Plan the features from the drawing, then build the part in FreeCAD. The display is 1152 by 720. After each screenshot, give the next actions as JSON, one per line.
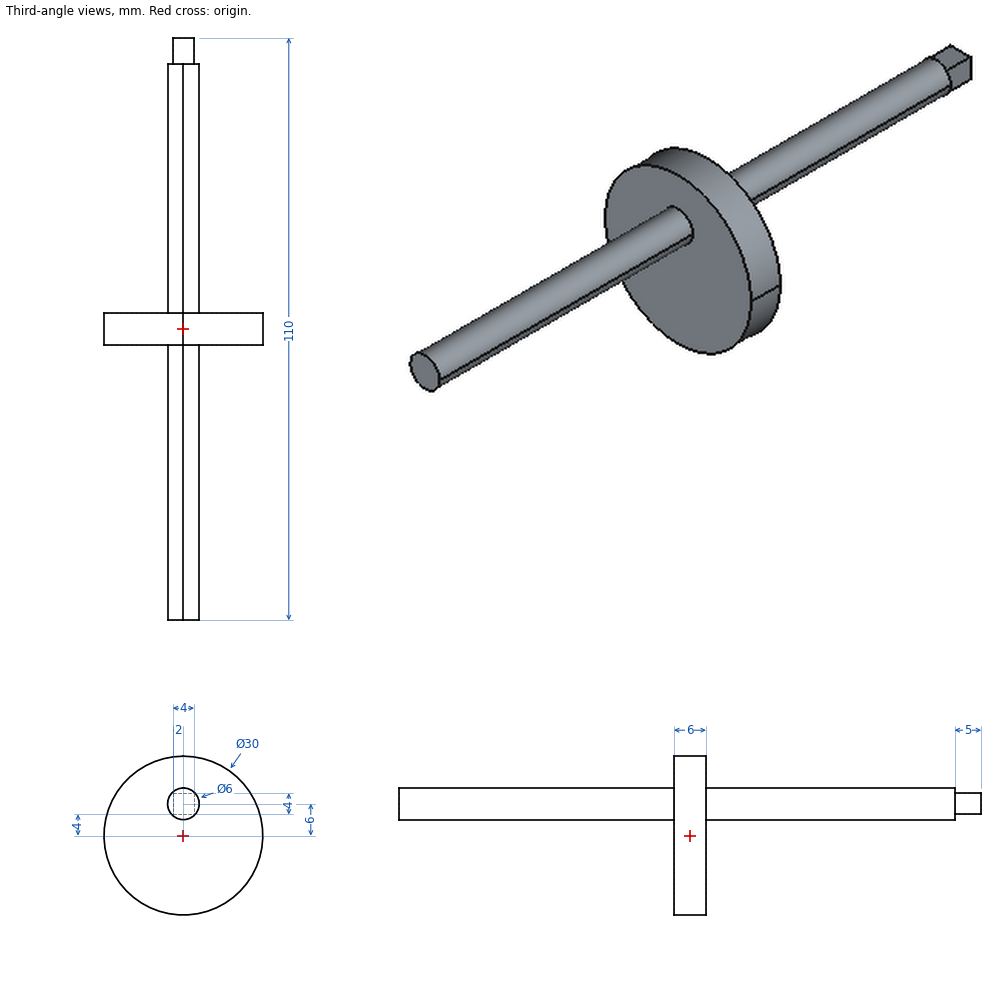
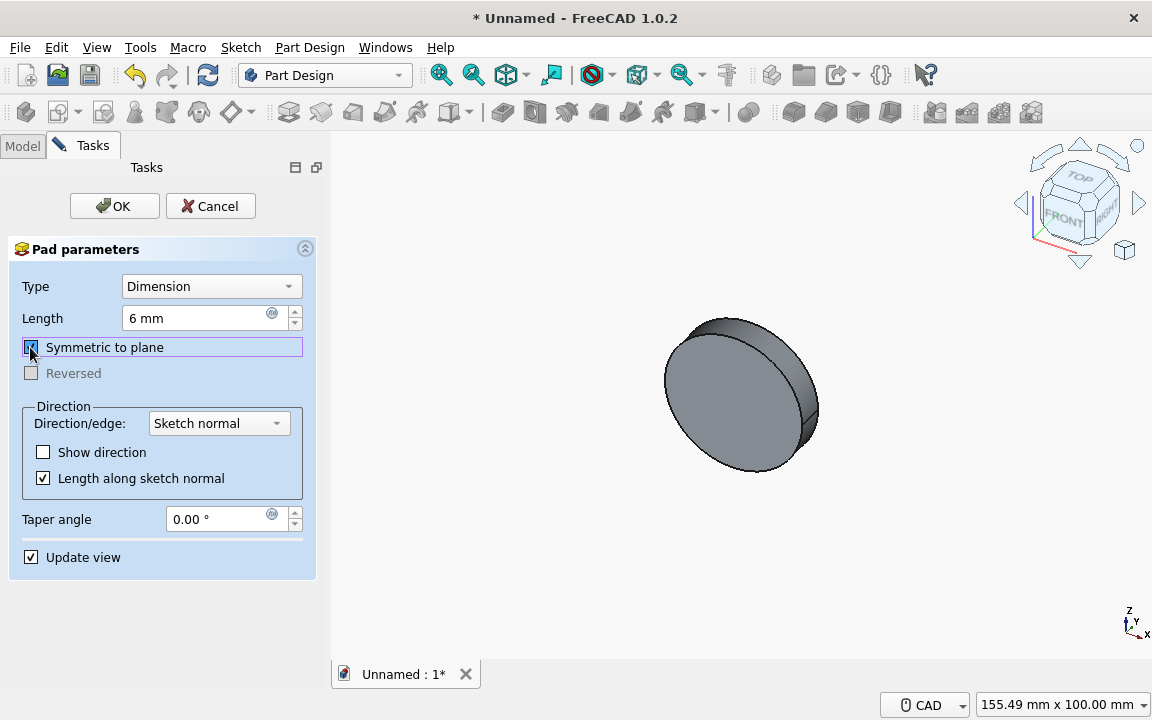
{"action": "left_click", "coordinate": [115, 206]}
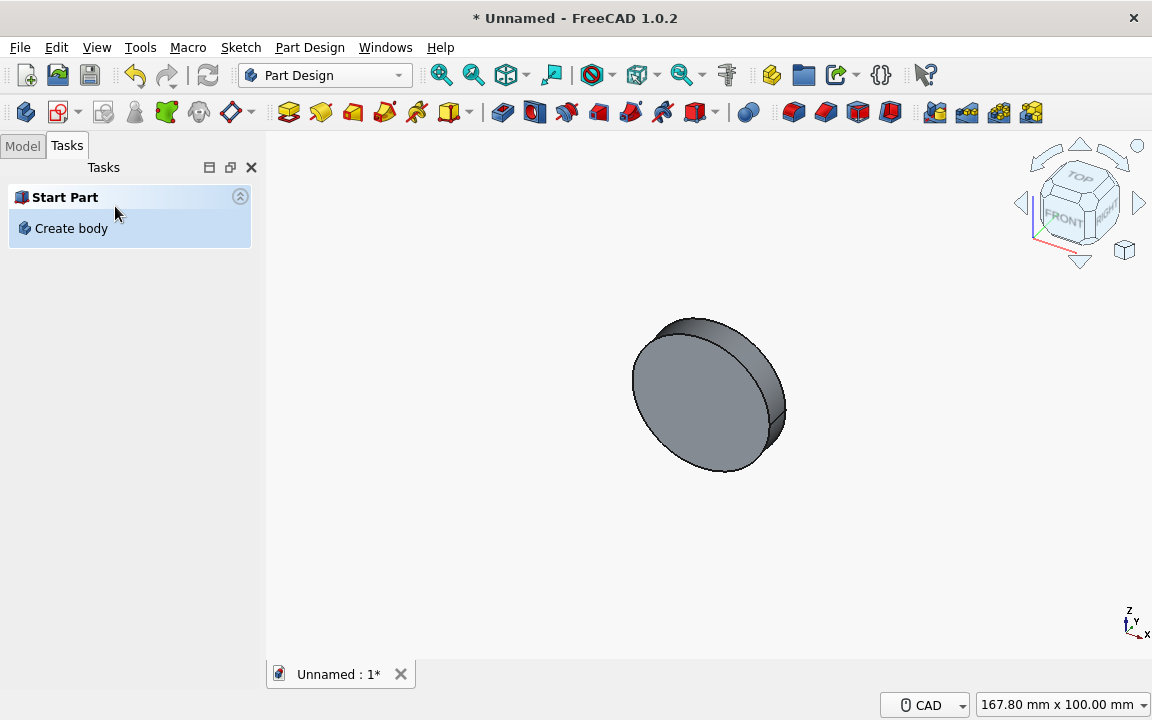
{"action": "key", "text": "v f"}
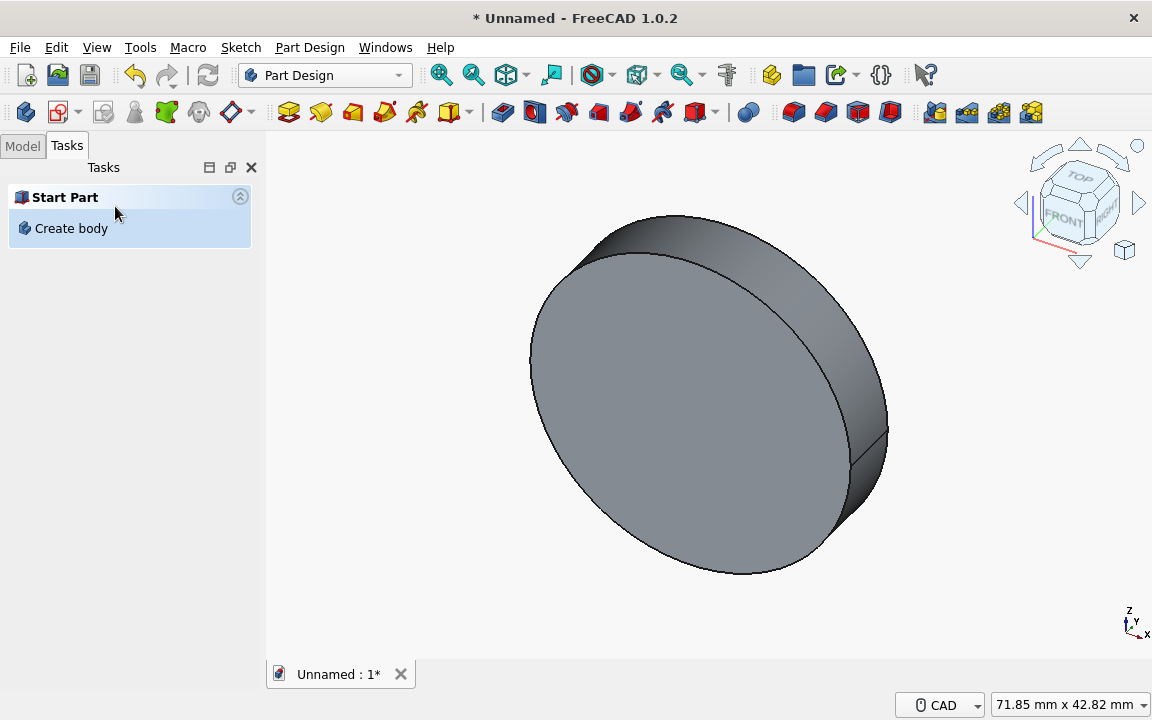
{"action": "left_click", "coordinate": [58, 112]}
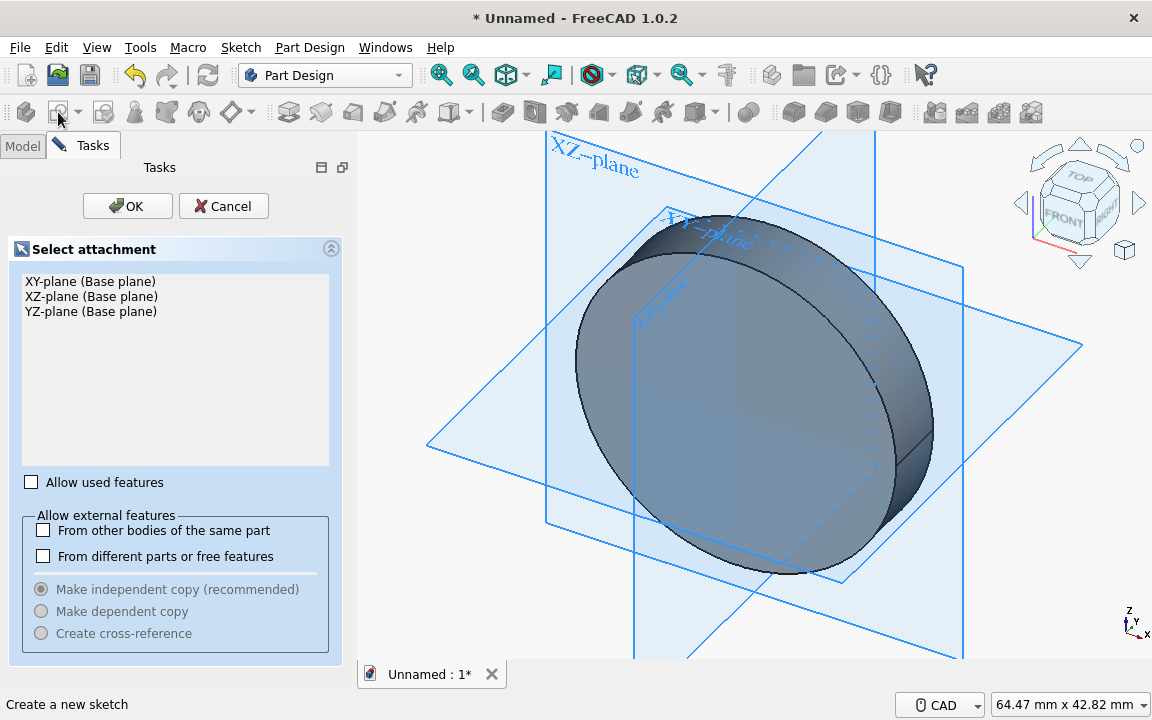
{"action": "left_click", "coordinate": [82, 296]}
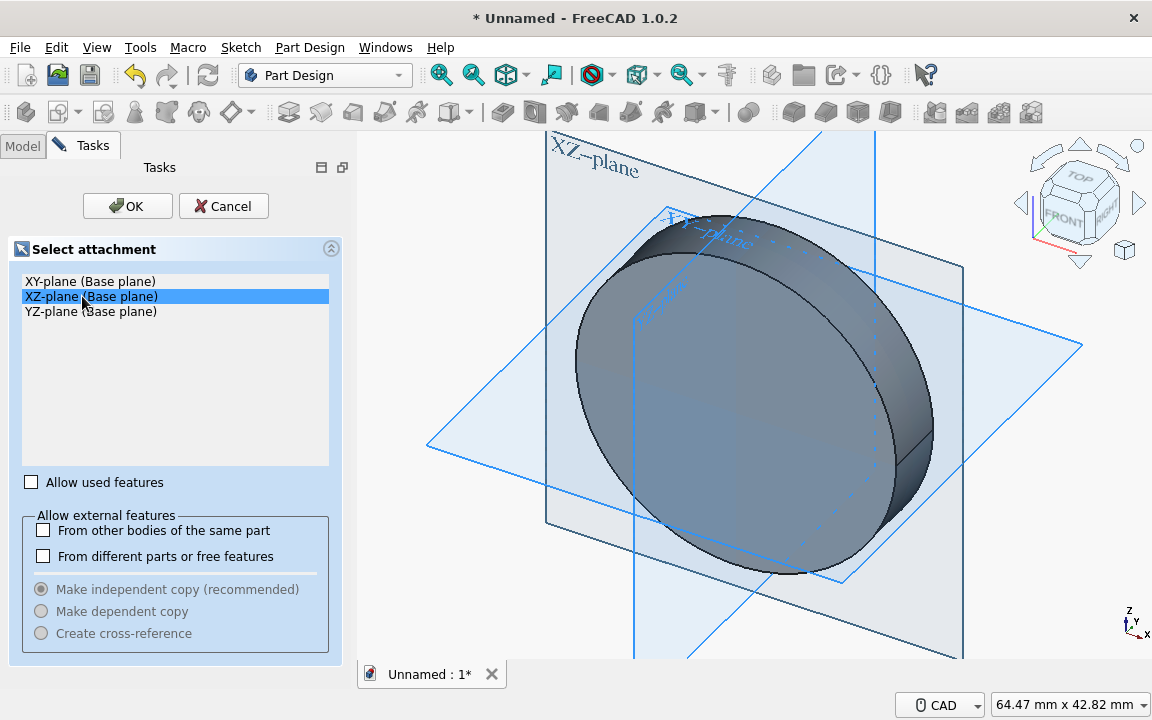
{"action": "left_click", "coordinate": [128, 206]}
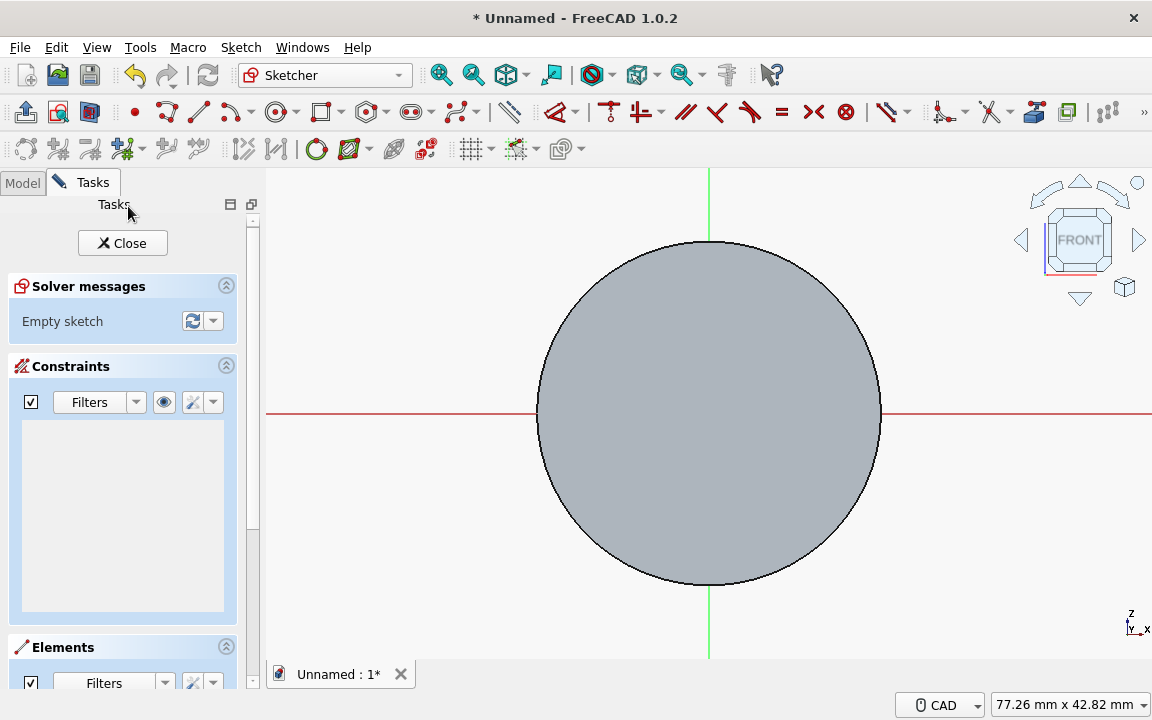
{"action": "key", "text": "q s"}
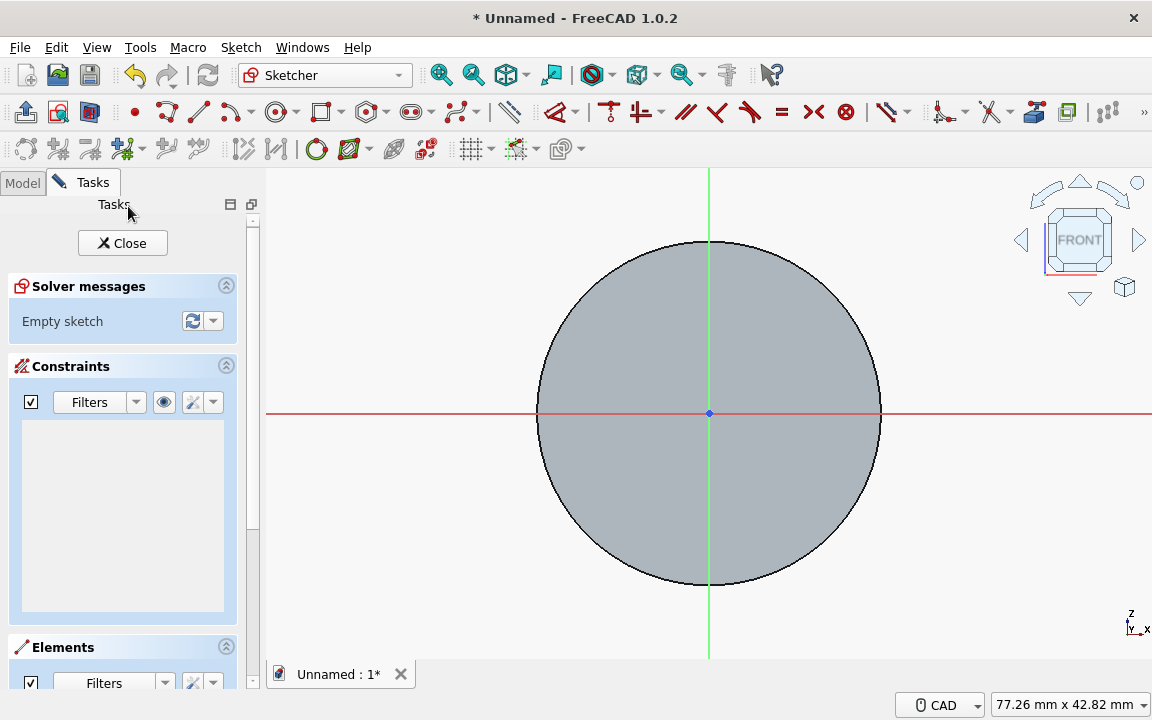
{"action": "scroll", "coordinate": [749, 332], "scroll_direction": "up", "scroll_amount": 5}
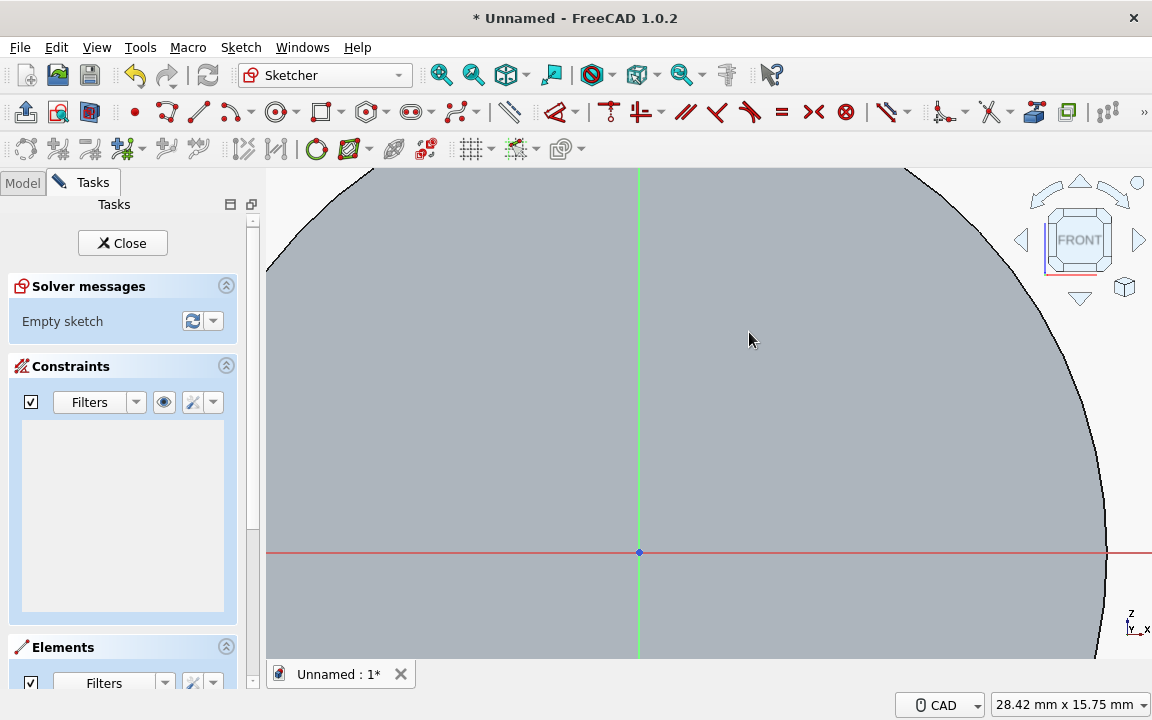
{"action": "key", "text": "g c"}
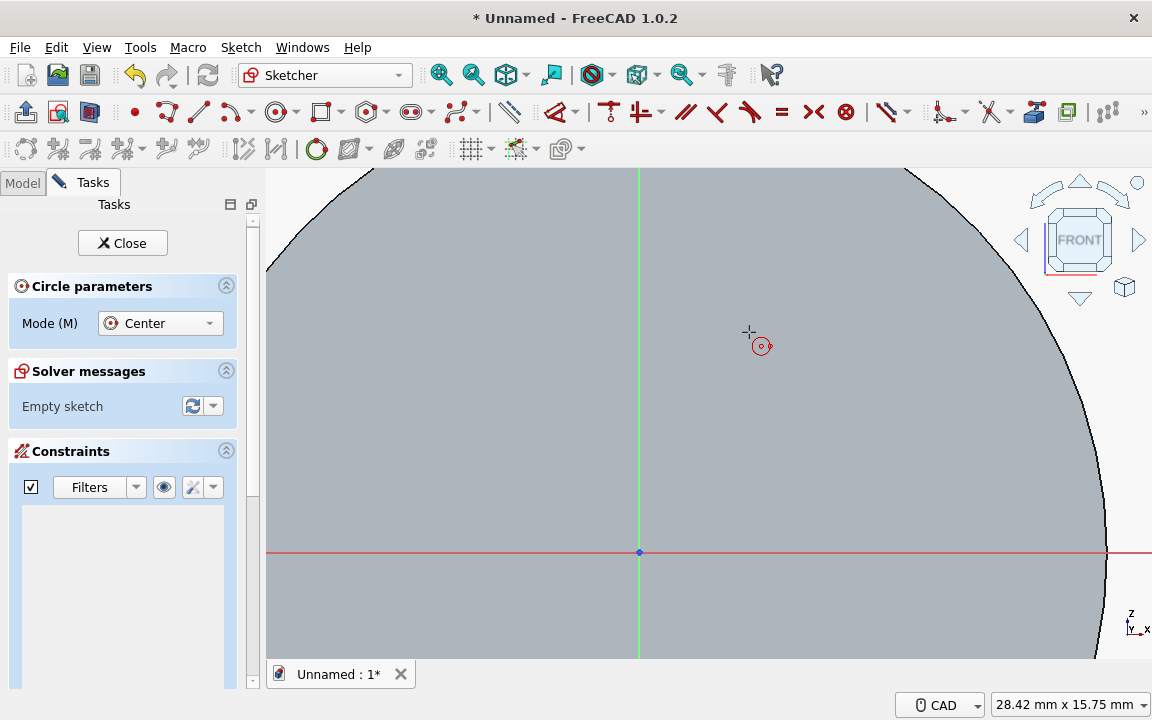
{"action": "left_click", "coordinate": [639, 366]}
{"action": "mouse_move", "coordinate": [705, 300]}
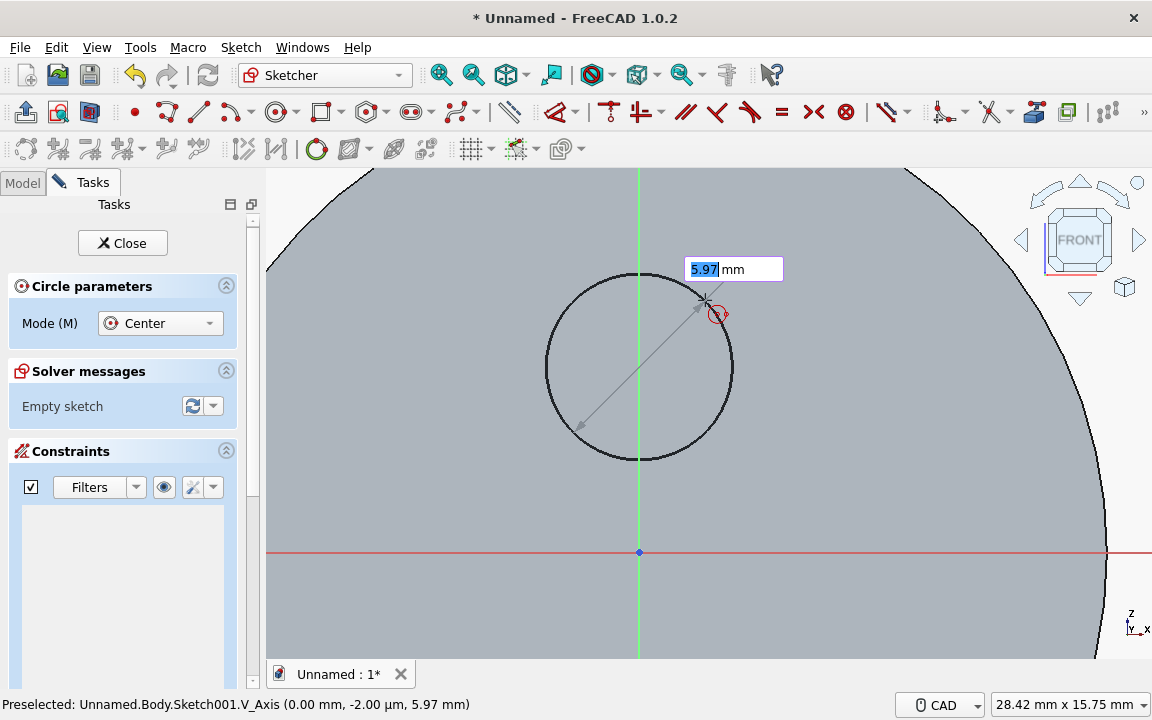
{"action": "type", "text": "6"}
{"action": "key", "text": "Return"}
{"action": "key", "text": "Escape"}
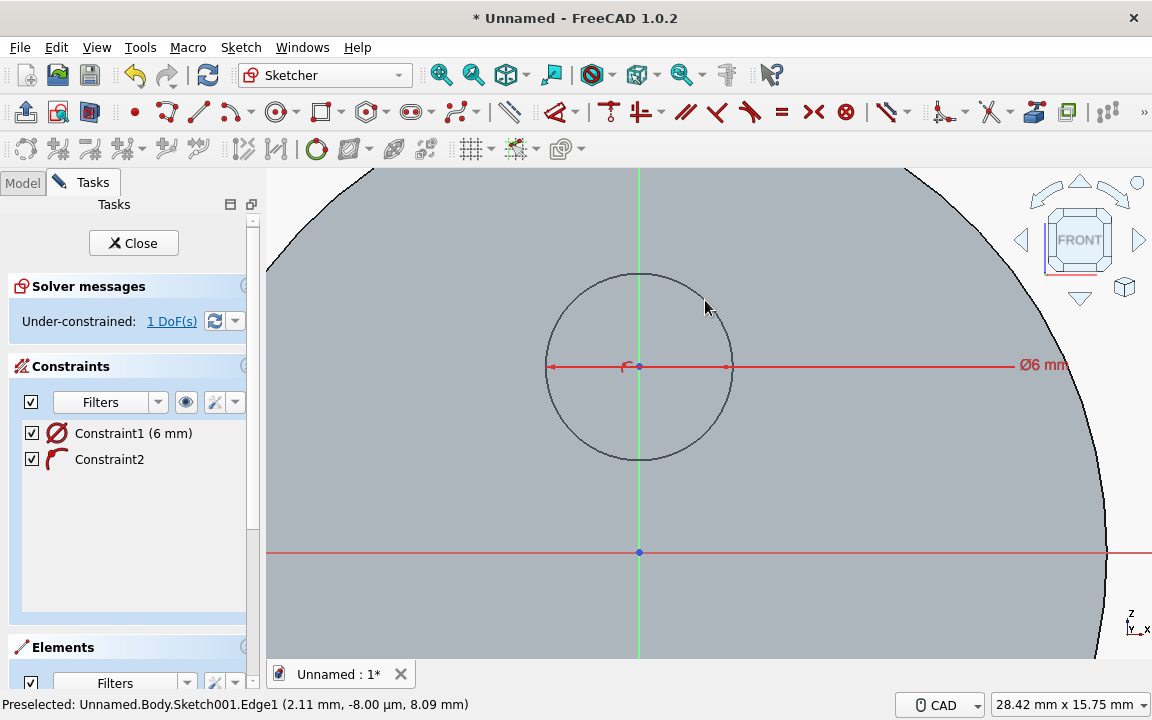
{"action": "left_click", "coordinate": [639, 367]}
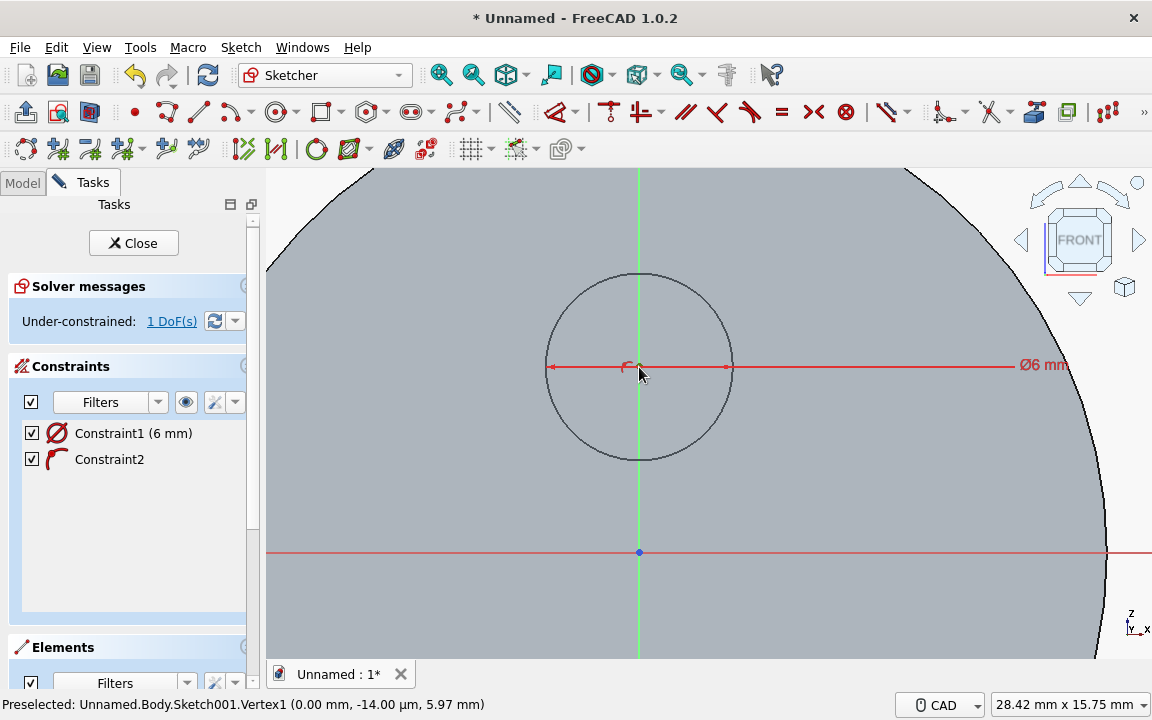
{"action": "key", "text": "i"}